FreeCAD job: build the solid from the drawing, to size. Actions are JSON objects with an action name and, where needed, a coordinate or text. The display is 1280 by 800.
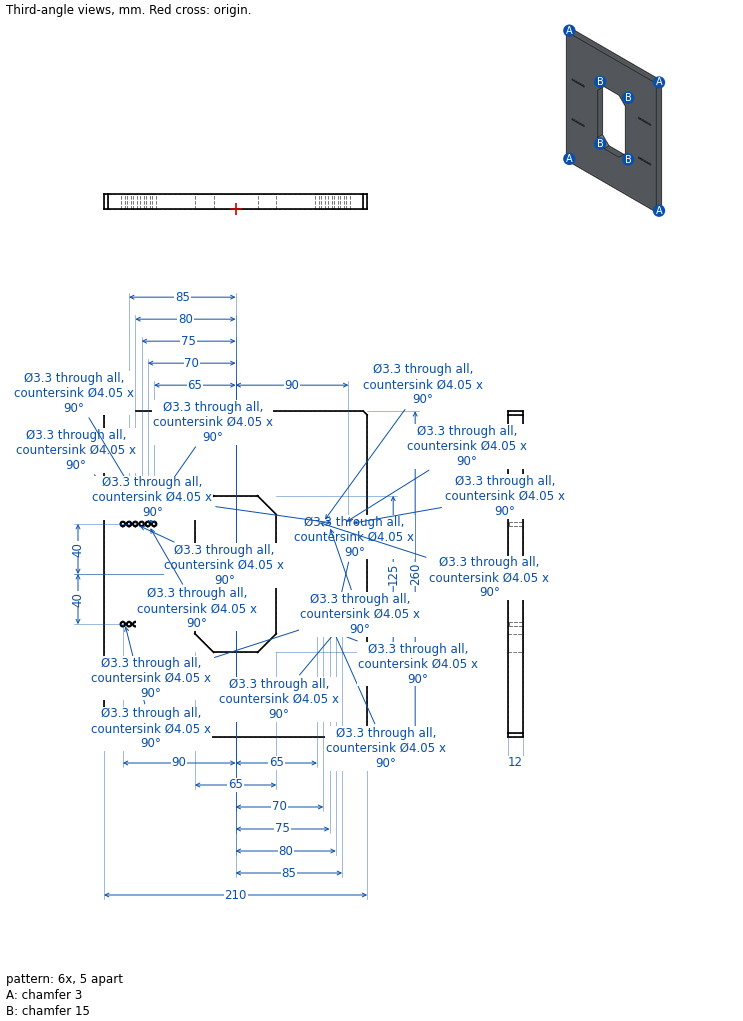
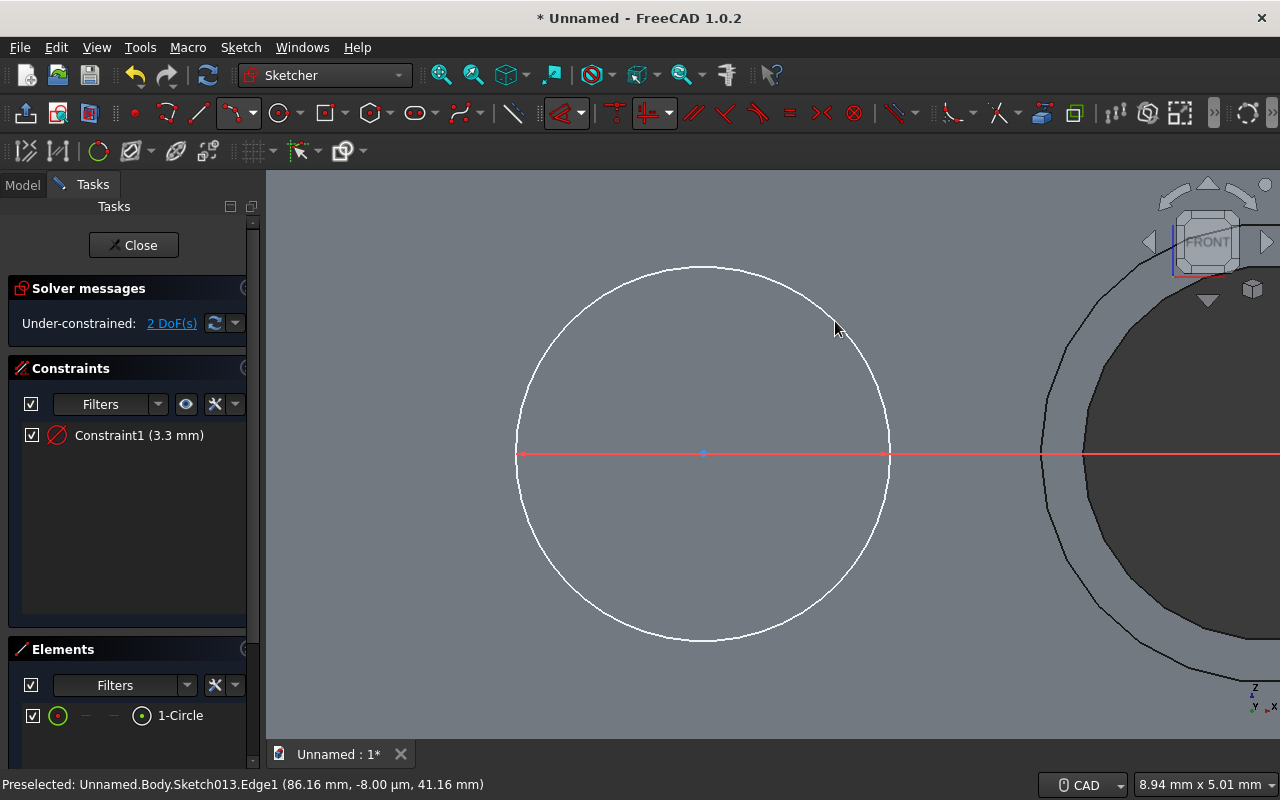
{"action": "left_click", "coordinate": [703, 454]}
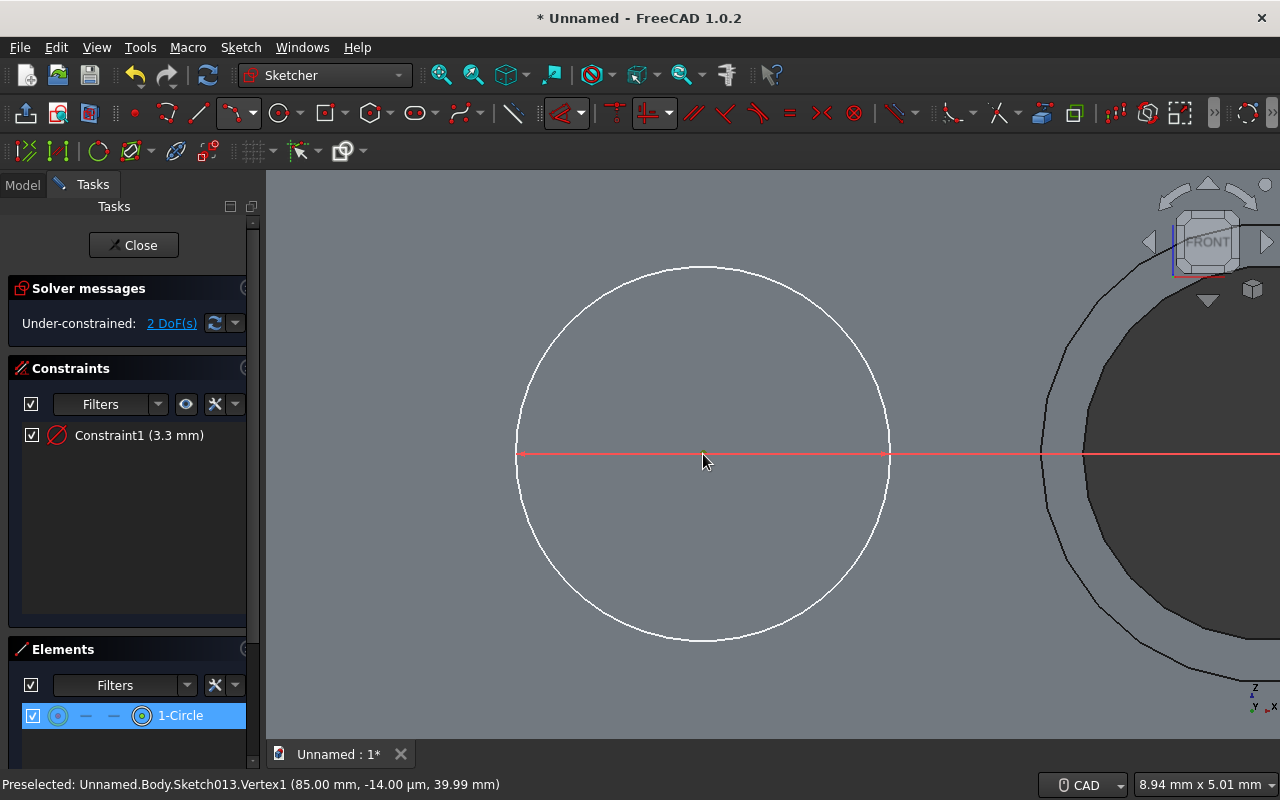
{"action": "left_click", "coordinate": [584, 114]}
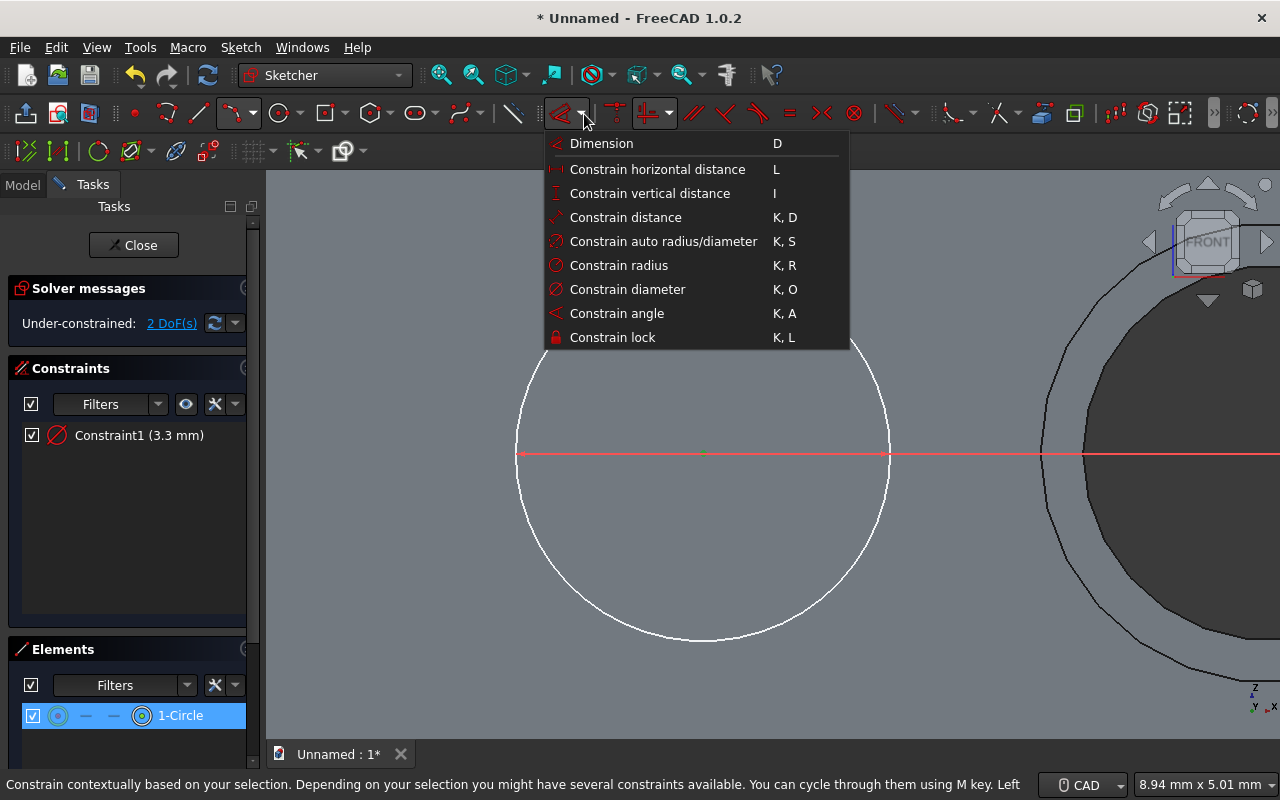
{"action": "left_click", "coordinate": [697, 169]}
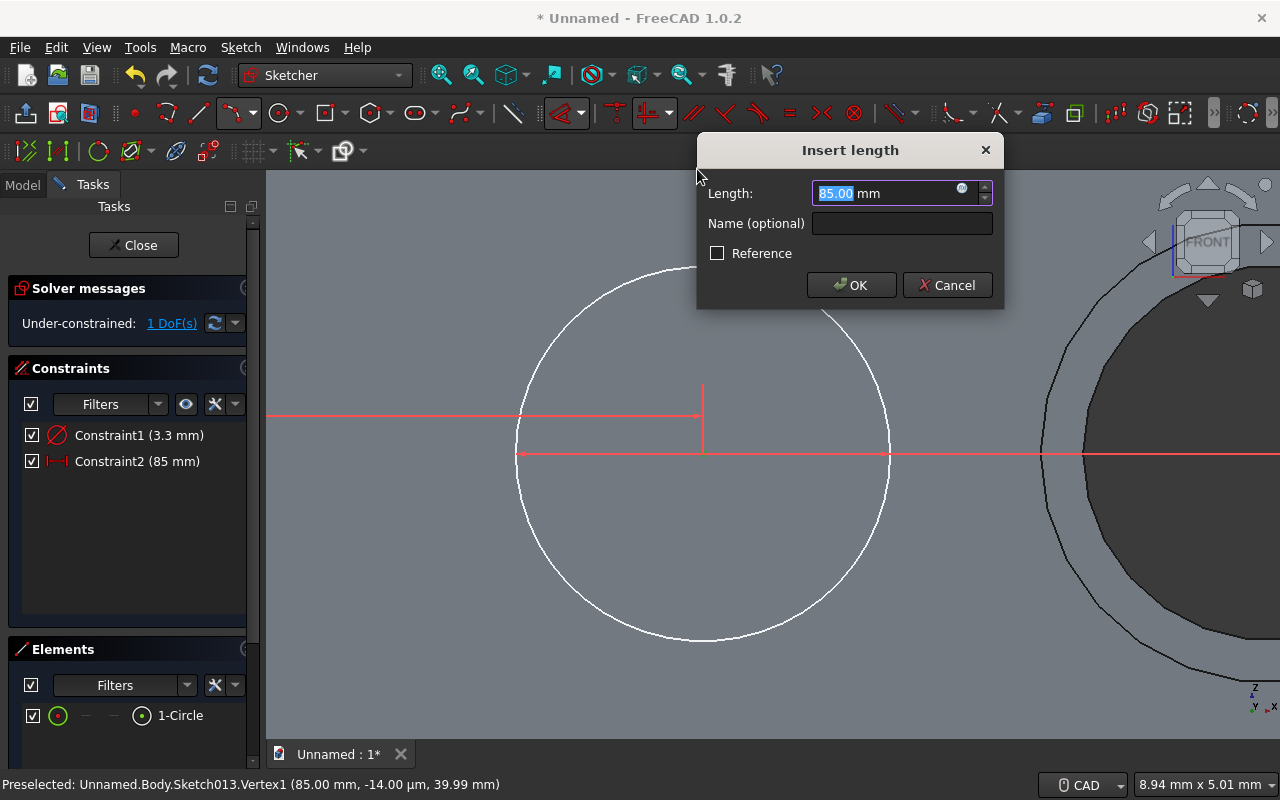
{"action": "type", "text": "85"}
{"action": "key", "text": "Return"}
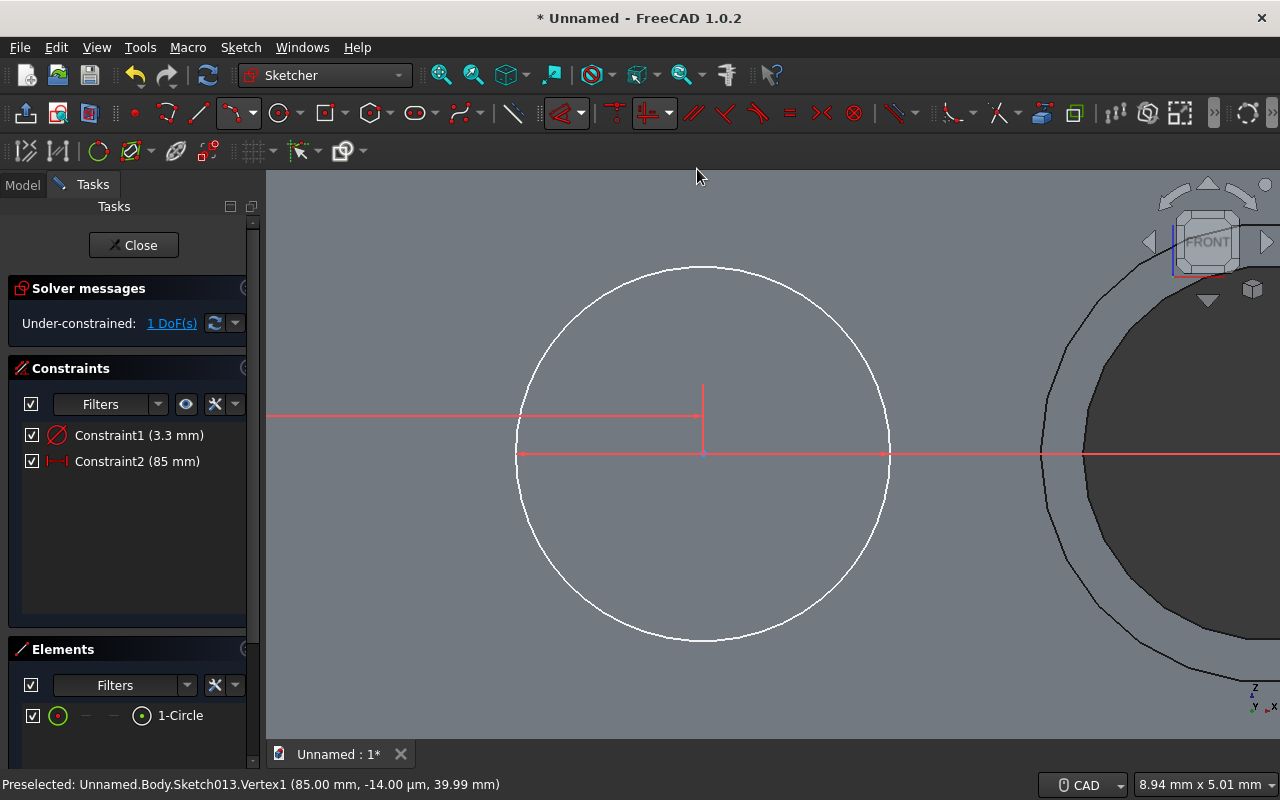
{"action": "left_click", "coordinate": [703, 454]}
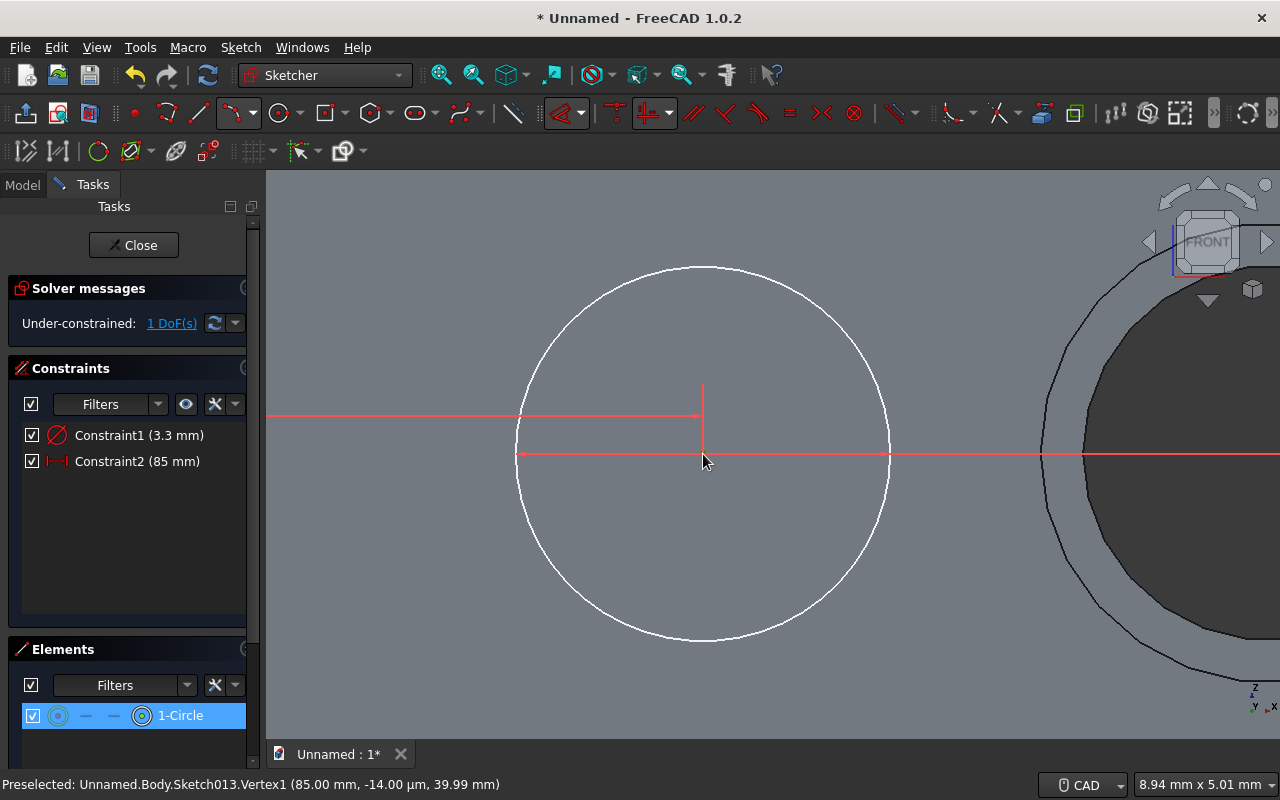
{"action": "left_click", "coordinate": [584, 114]}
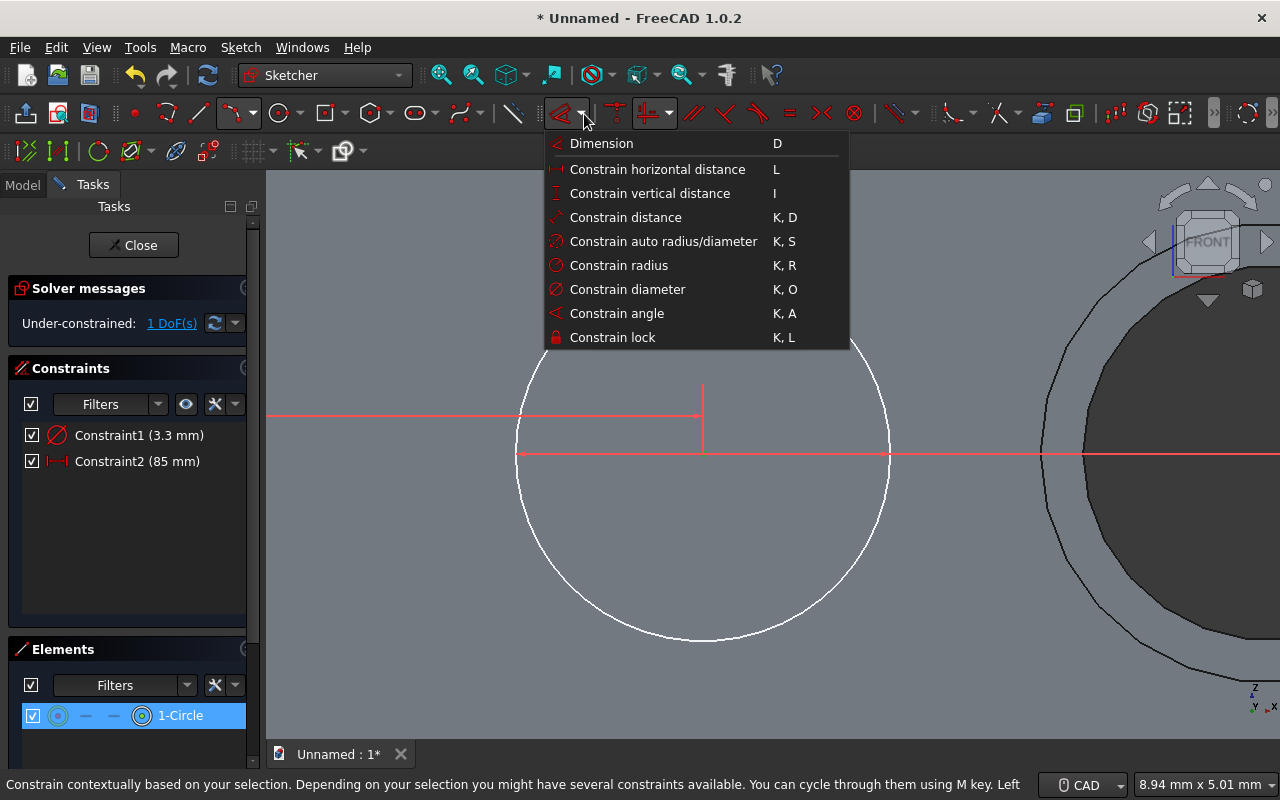
{"action": "left_click", "coordinate": [697, 193]}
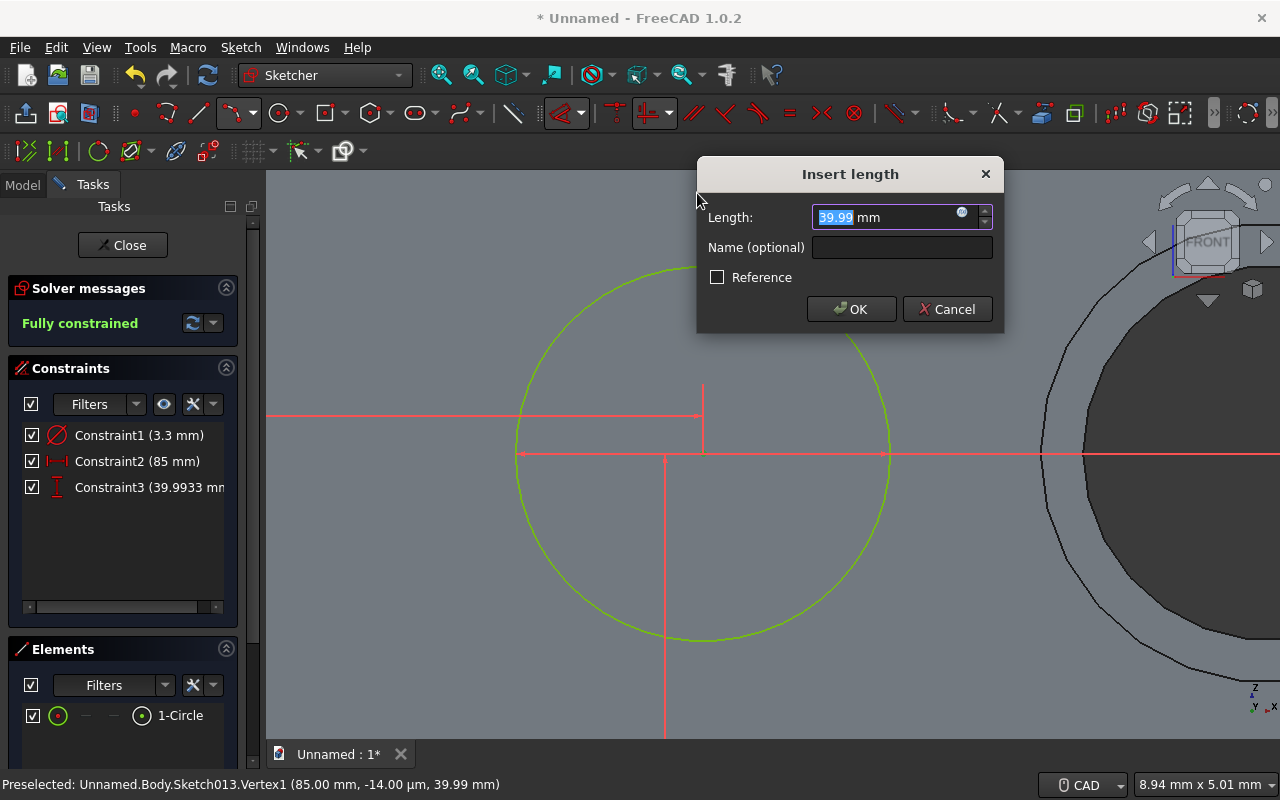
{"action": "type", "text": "40"}
{"action": "key", "text": "Return"}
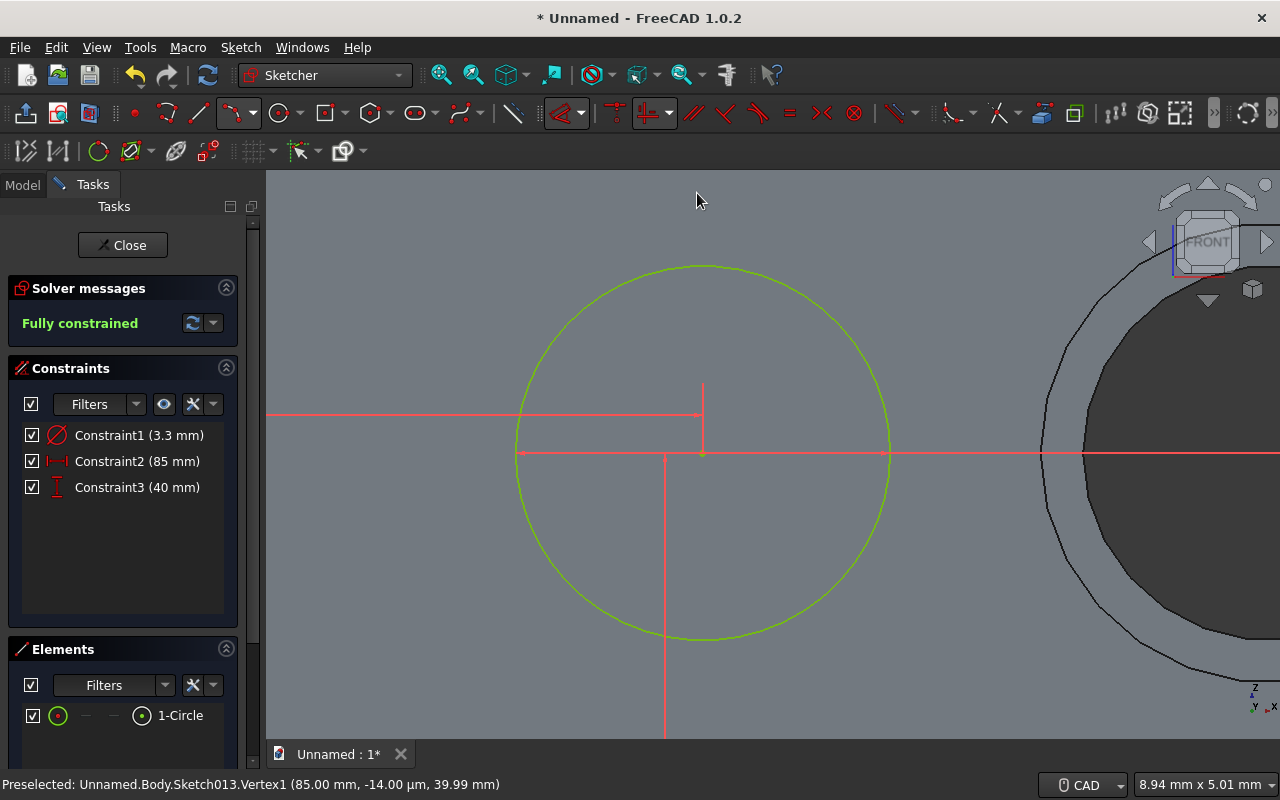
{"action": "left_click", "coordinate": [123, 245]}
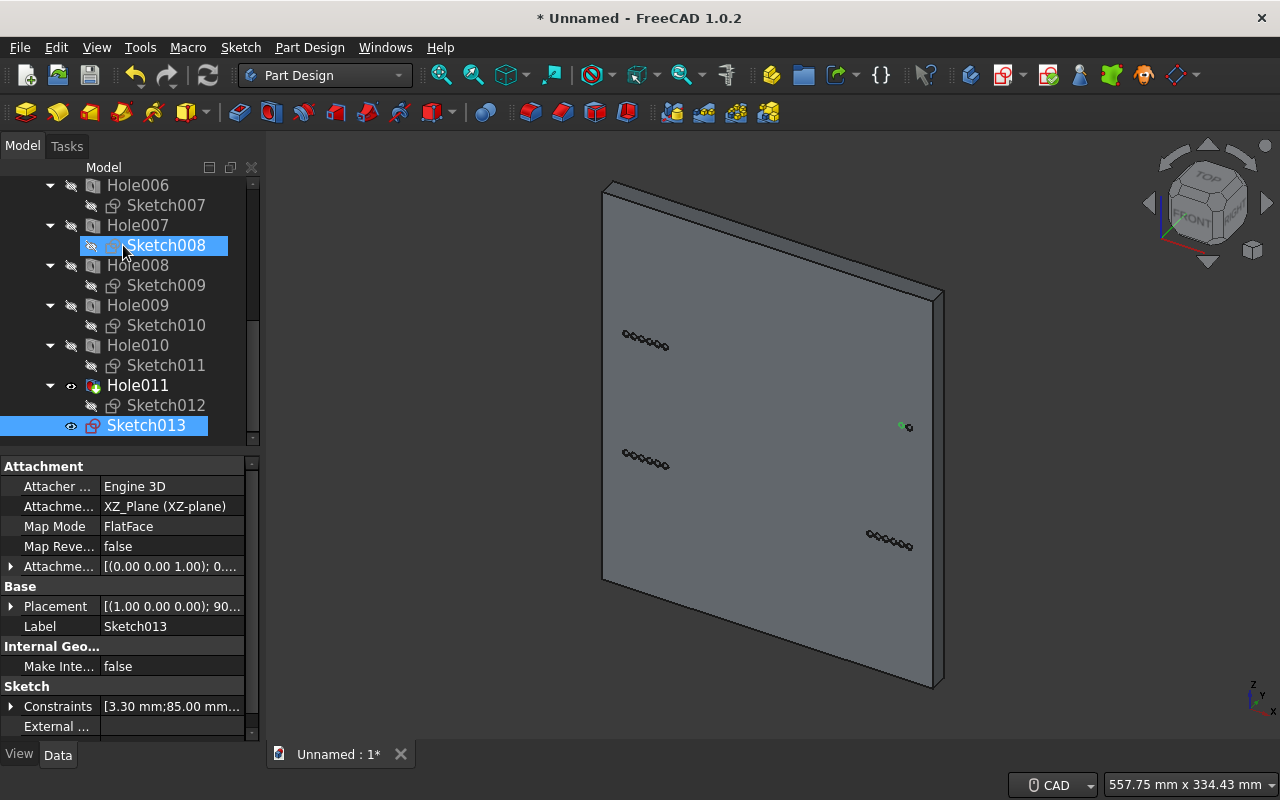
{"action": "left_click", "coordinate": [272, 112]}